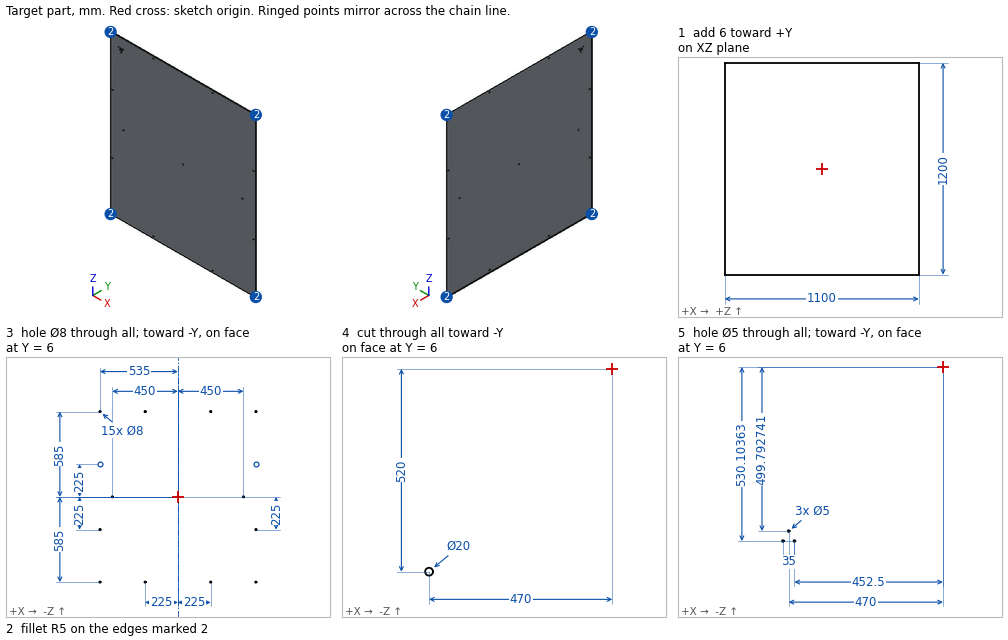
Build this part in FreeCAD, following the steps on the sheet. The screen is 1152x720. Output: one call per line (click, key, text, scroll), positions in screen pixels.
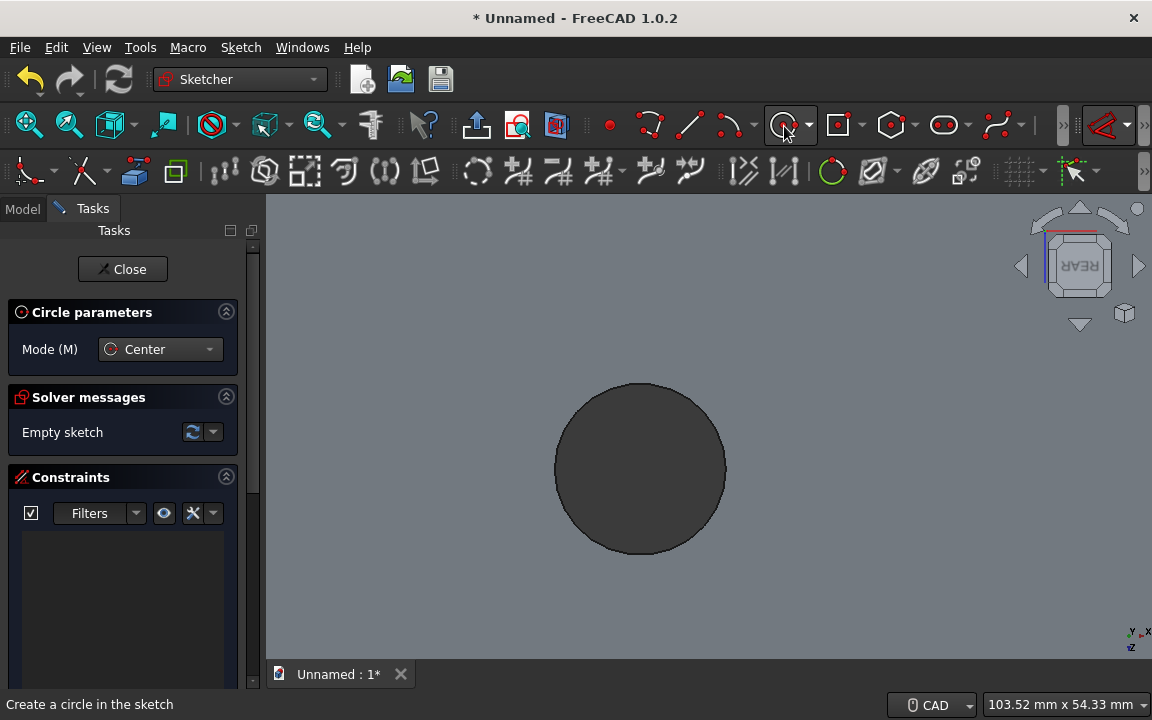
click(640, 296)
move(655, 281)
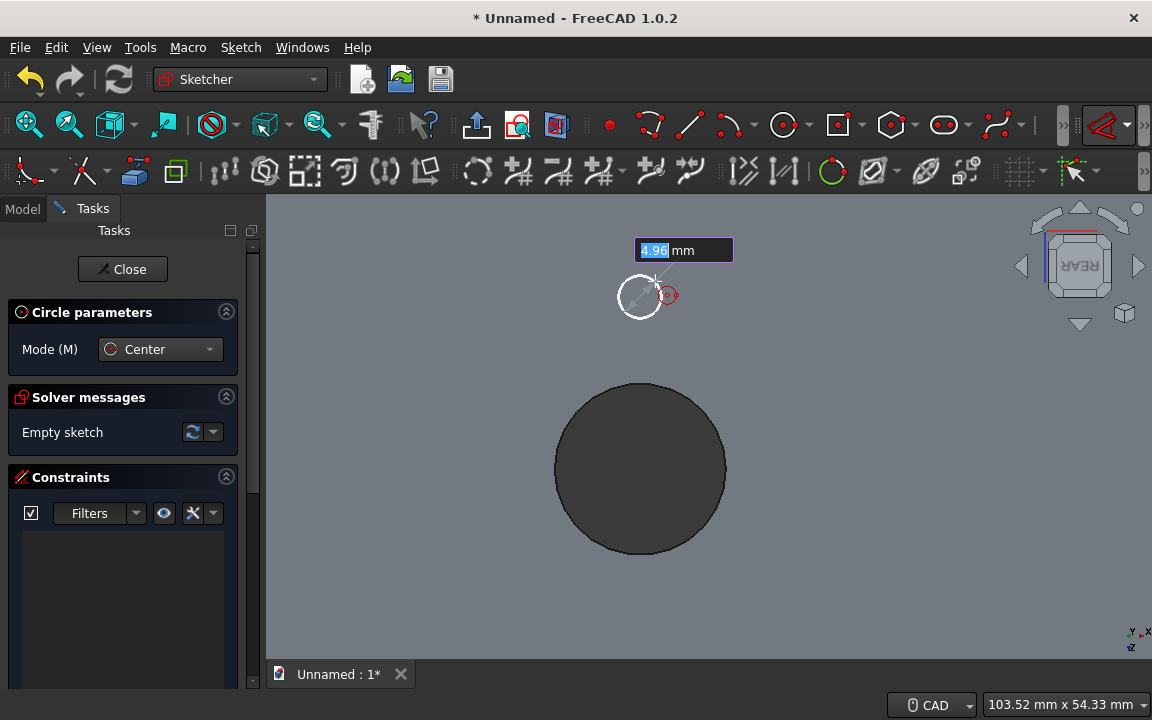
text(5)
key(Return)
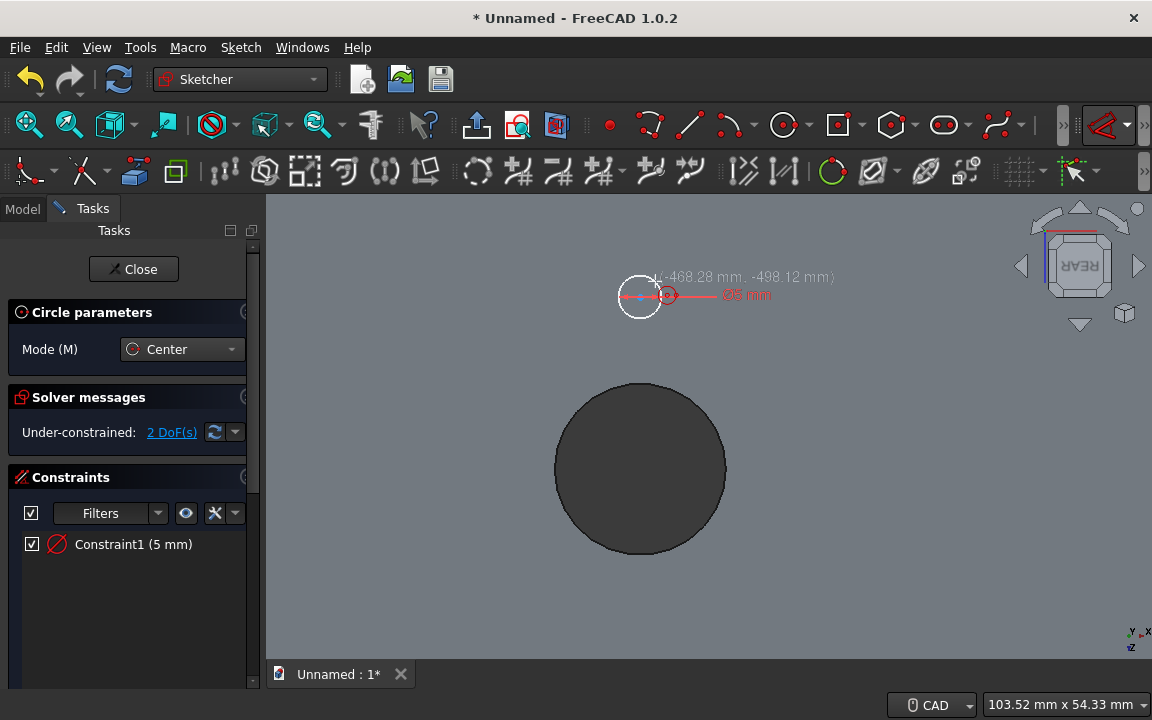
click(790, 556)
move(805, 541)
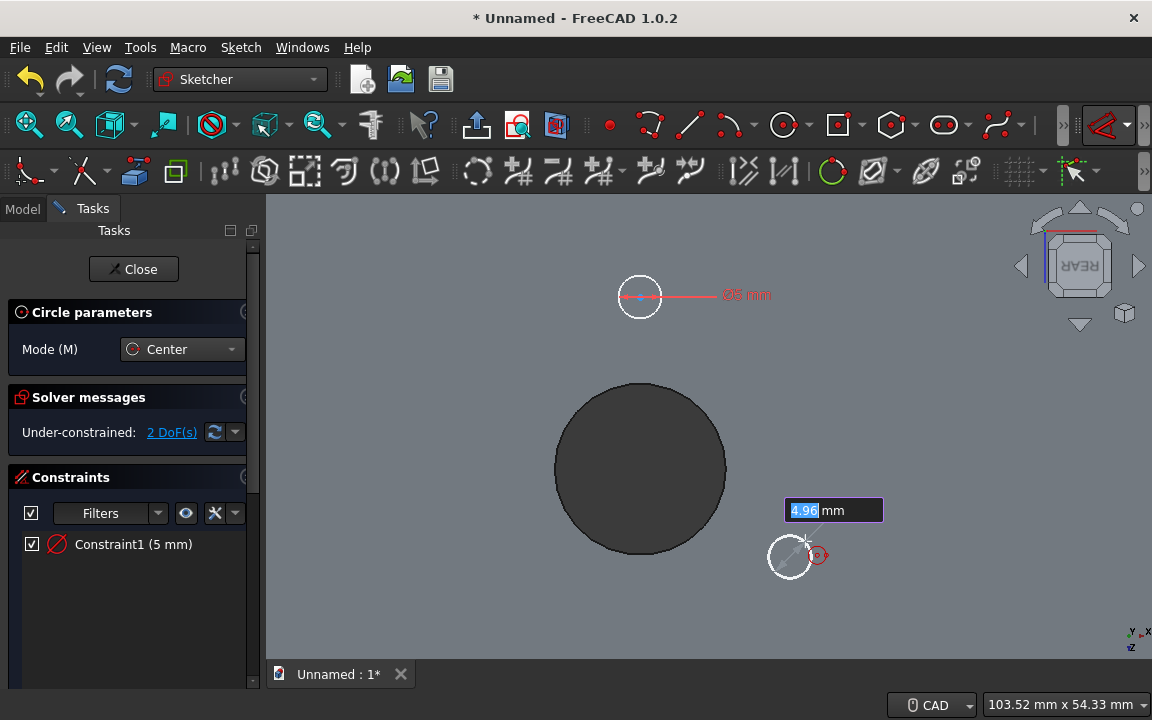
text(5)
key(Return)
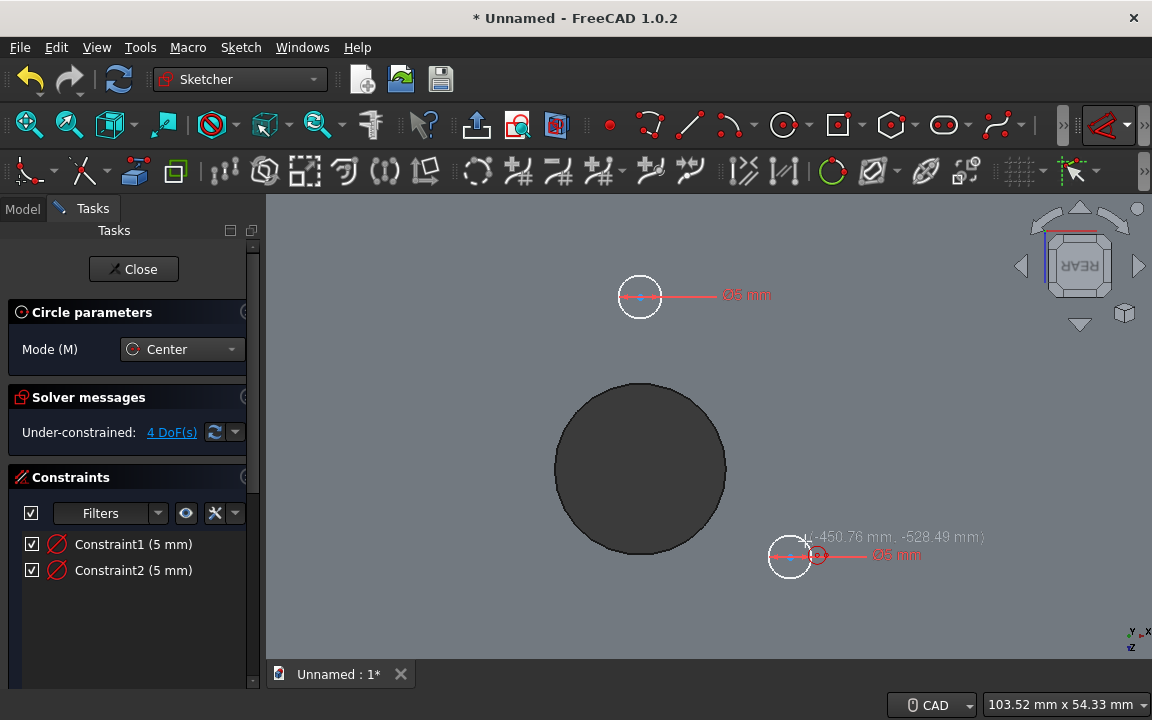
click(491, 556)
move(506, 541)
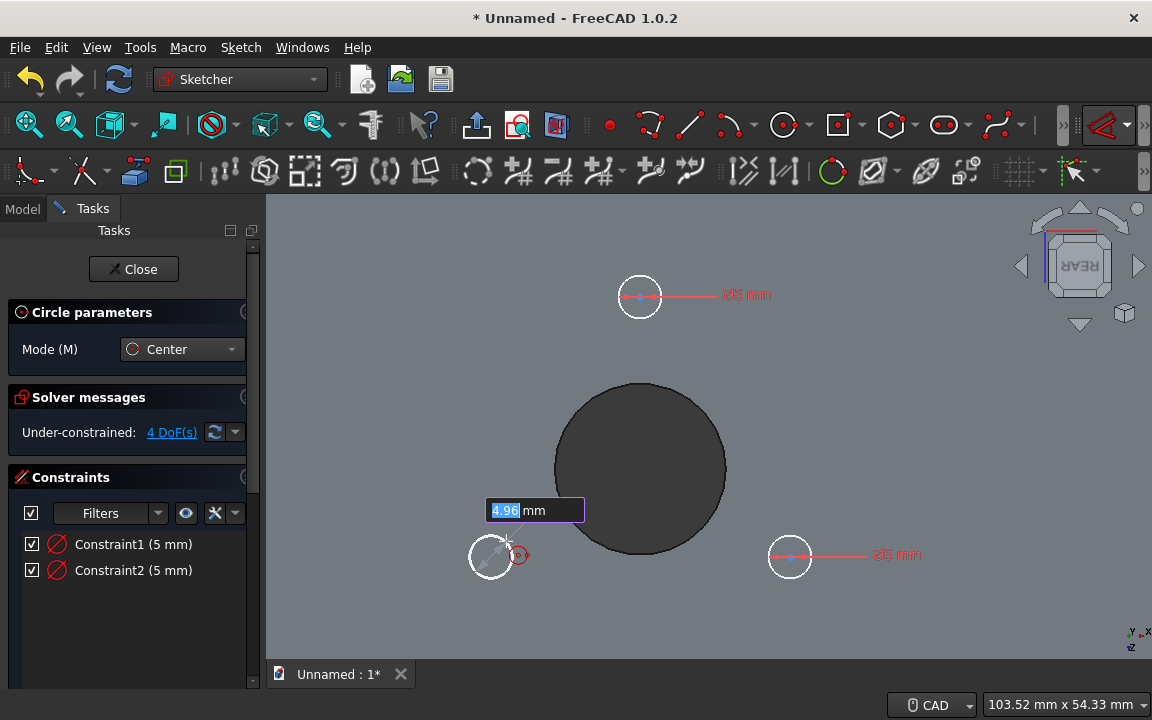
text(5)
key(Return)
key(Escape)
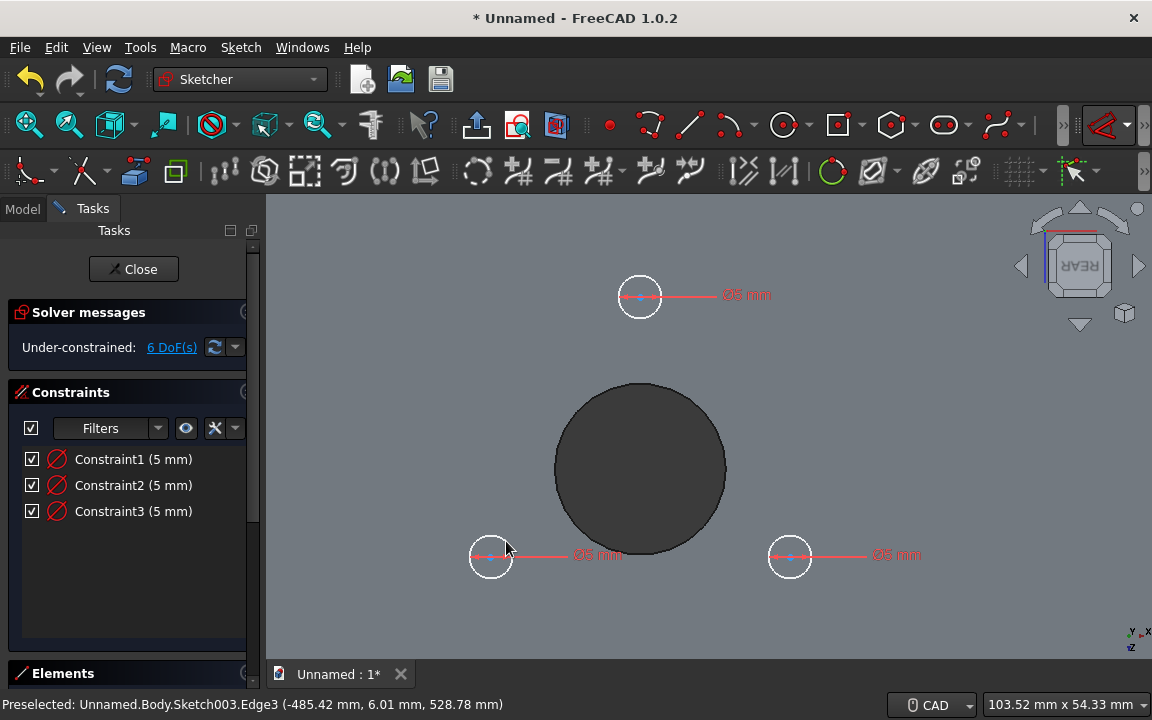
click(790, 557)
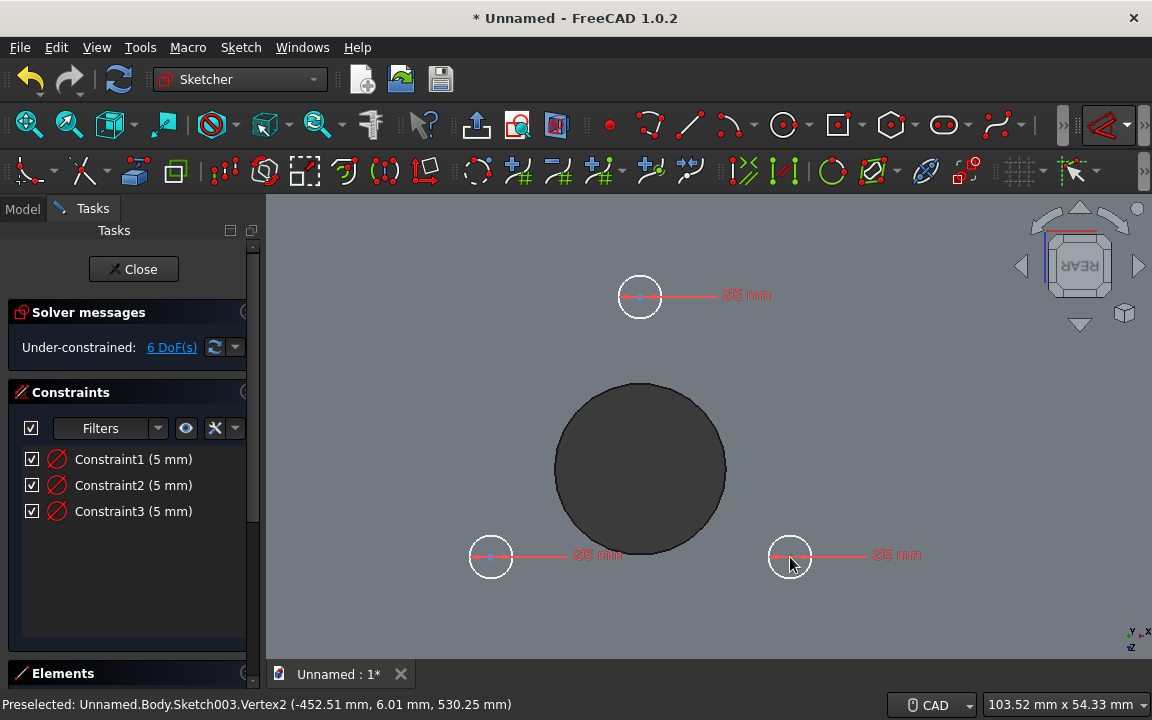
click(491, 557)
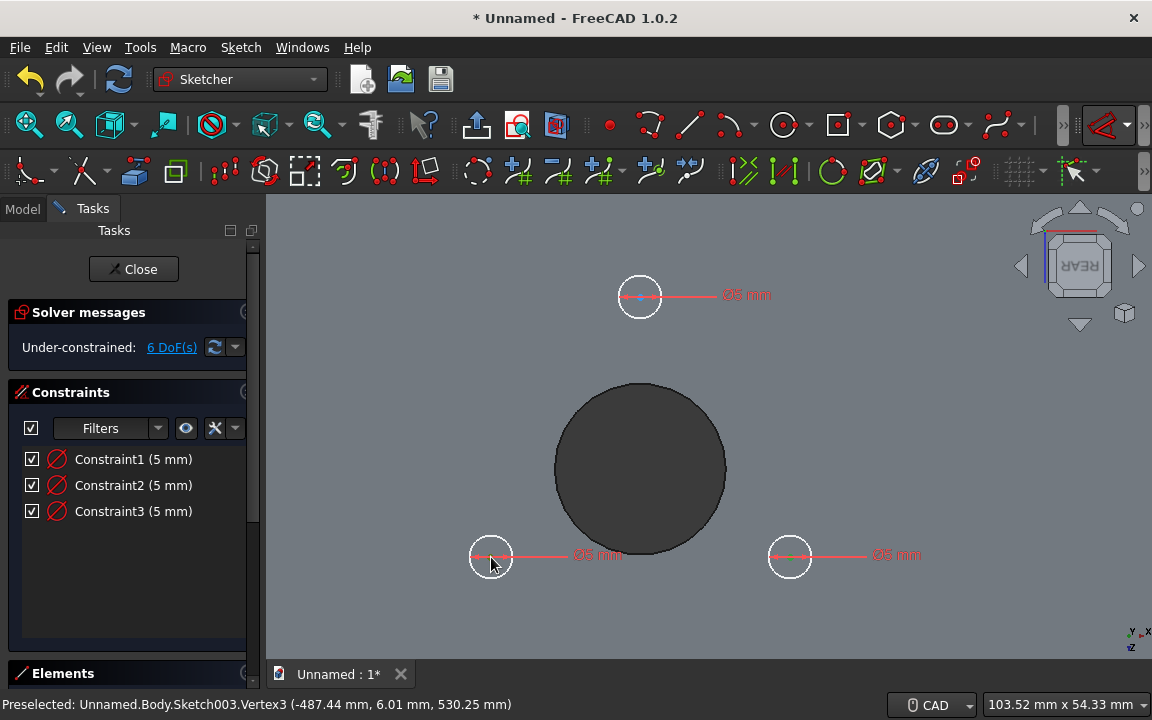
key(h)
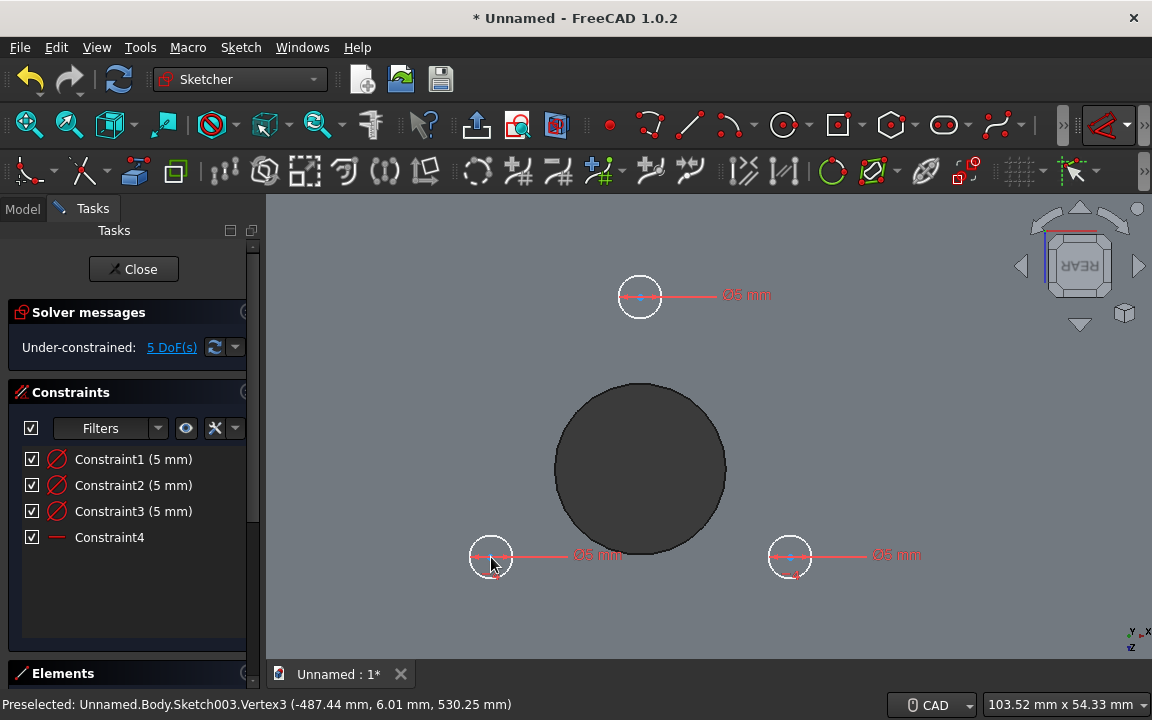
click(640, 297)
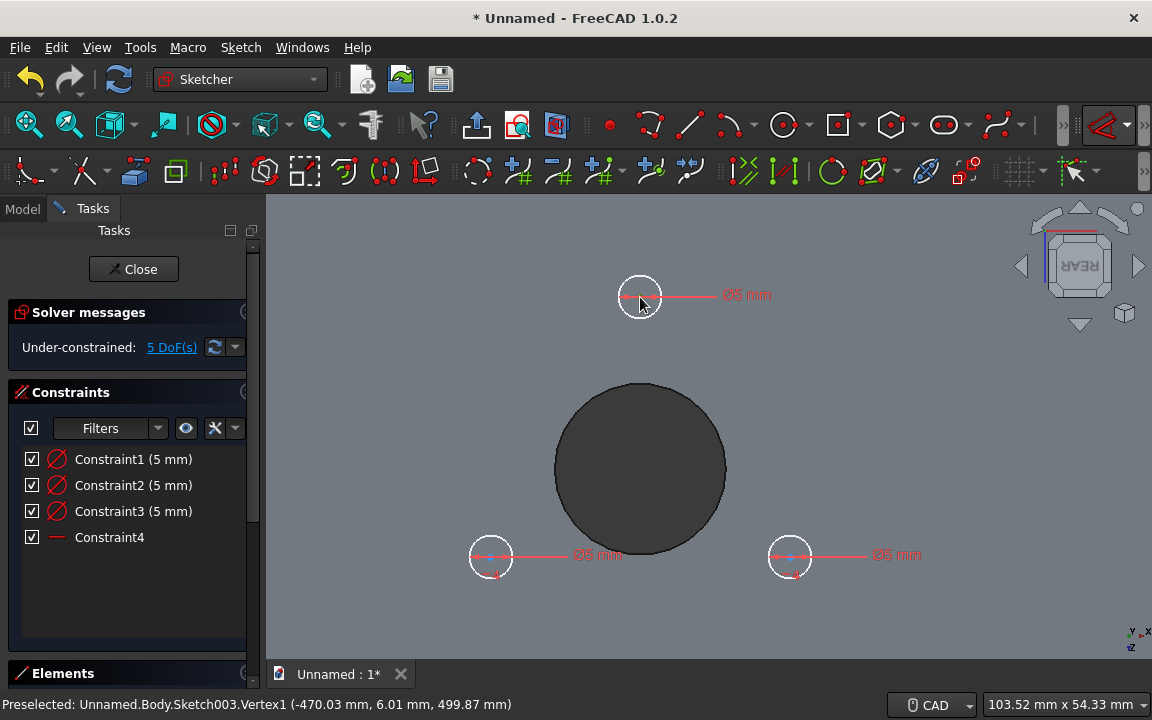
click(1130, 126)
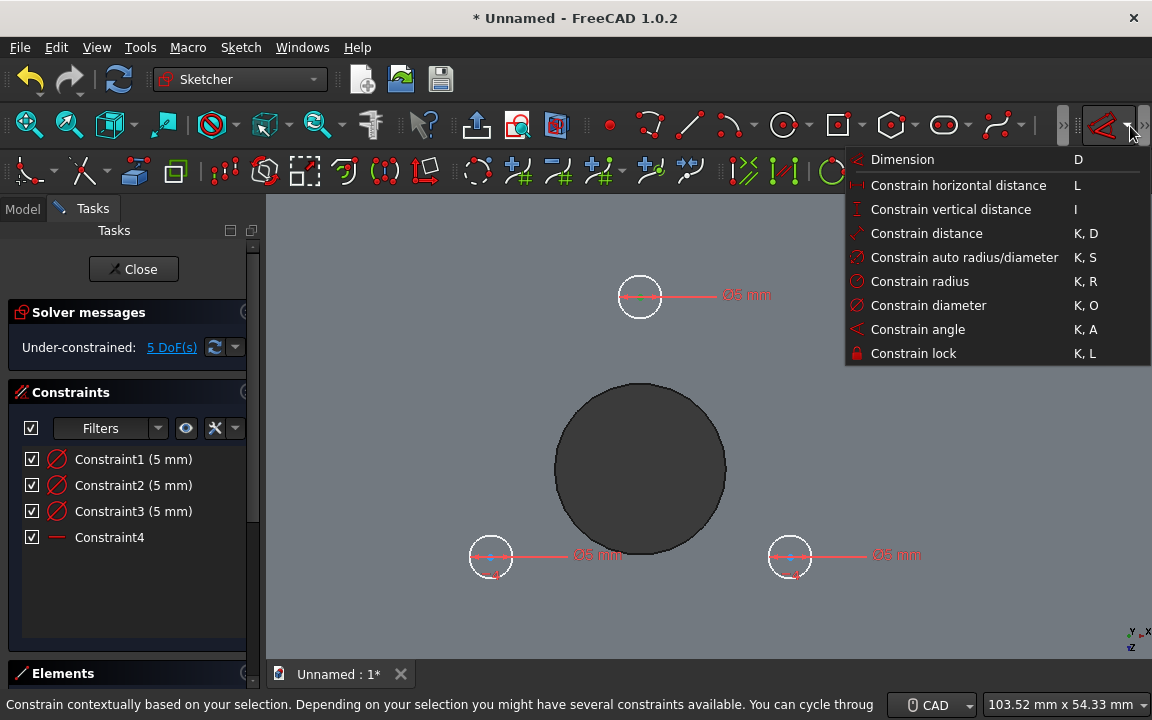
click(998, 185)